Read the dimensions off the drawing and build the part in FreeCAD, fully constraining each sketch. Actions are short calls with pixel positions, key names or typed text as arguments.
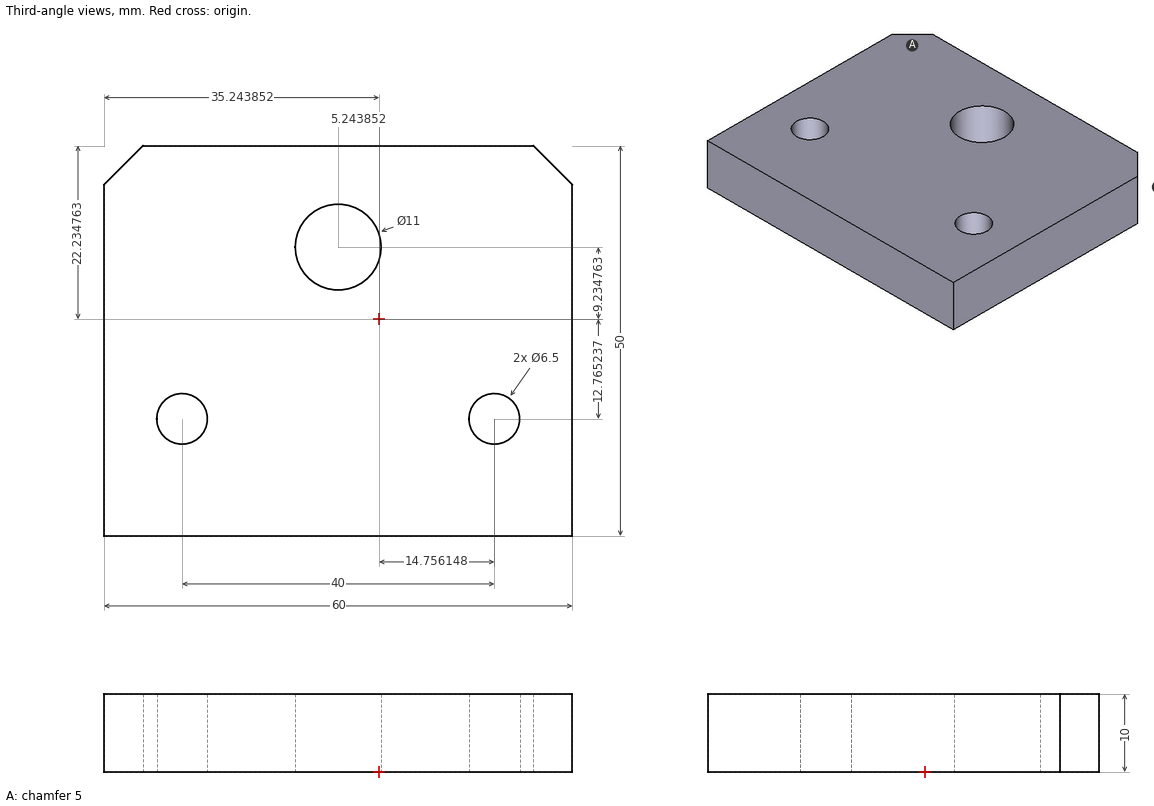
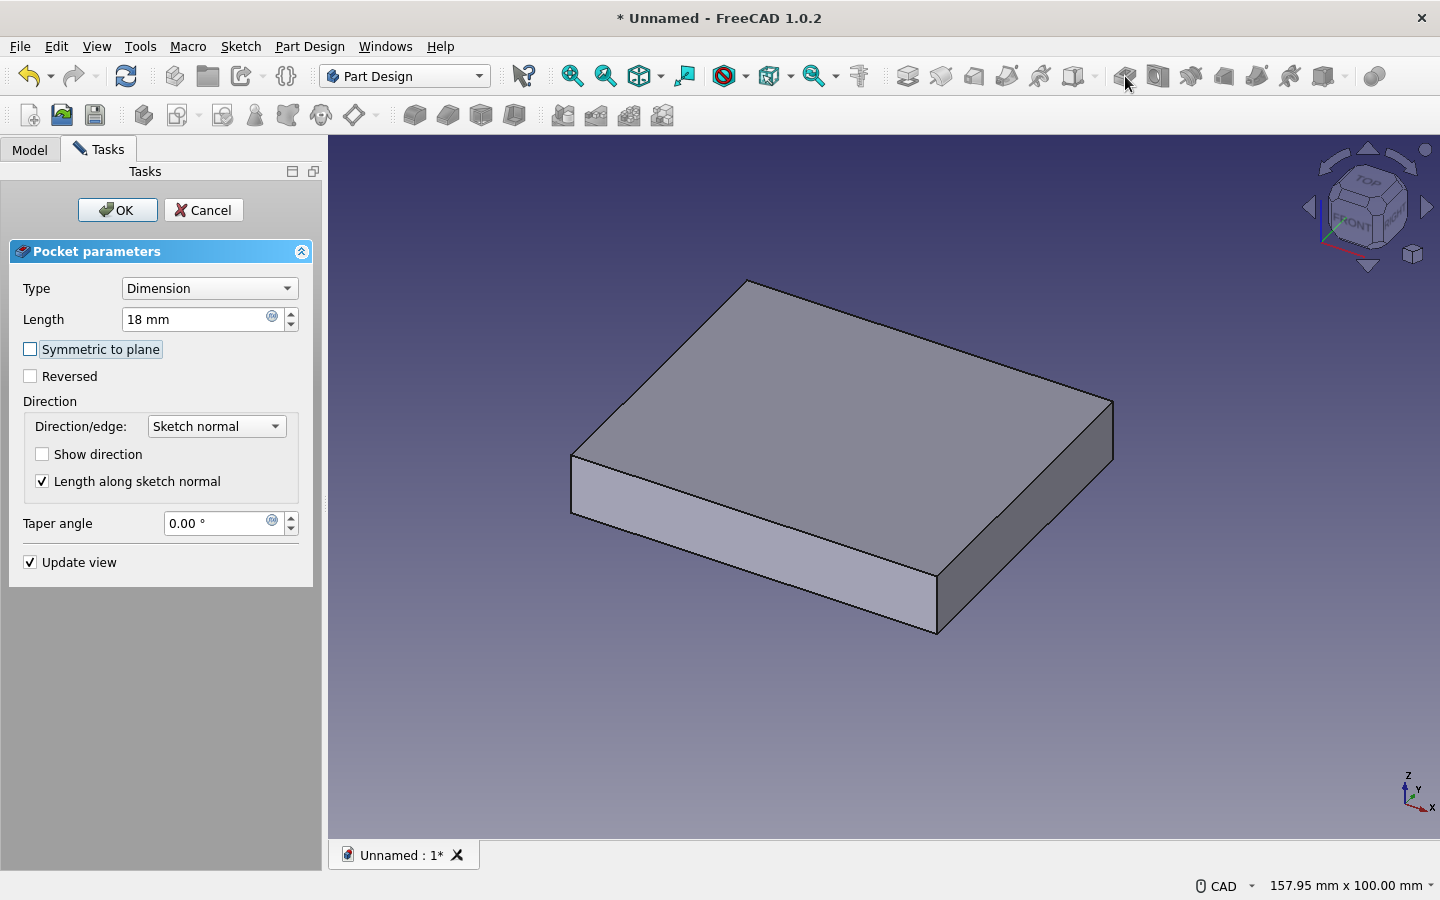
click(31, 376)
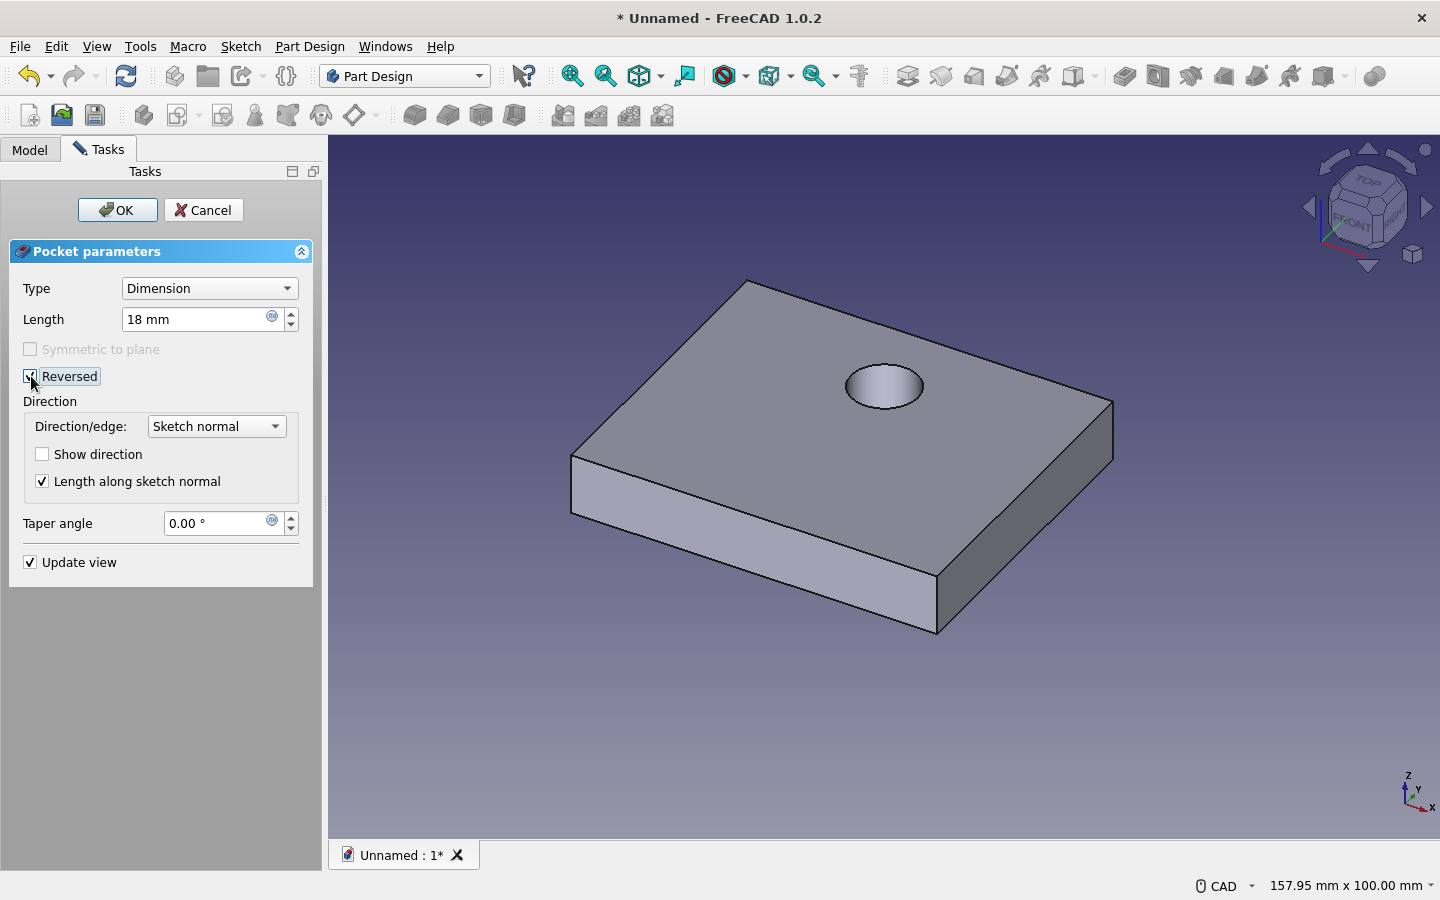
click(118, 210)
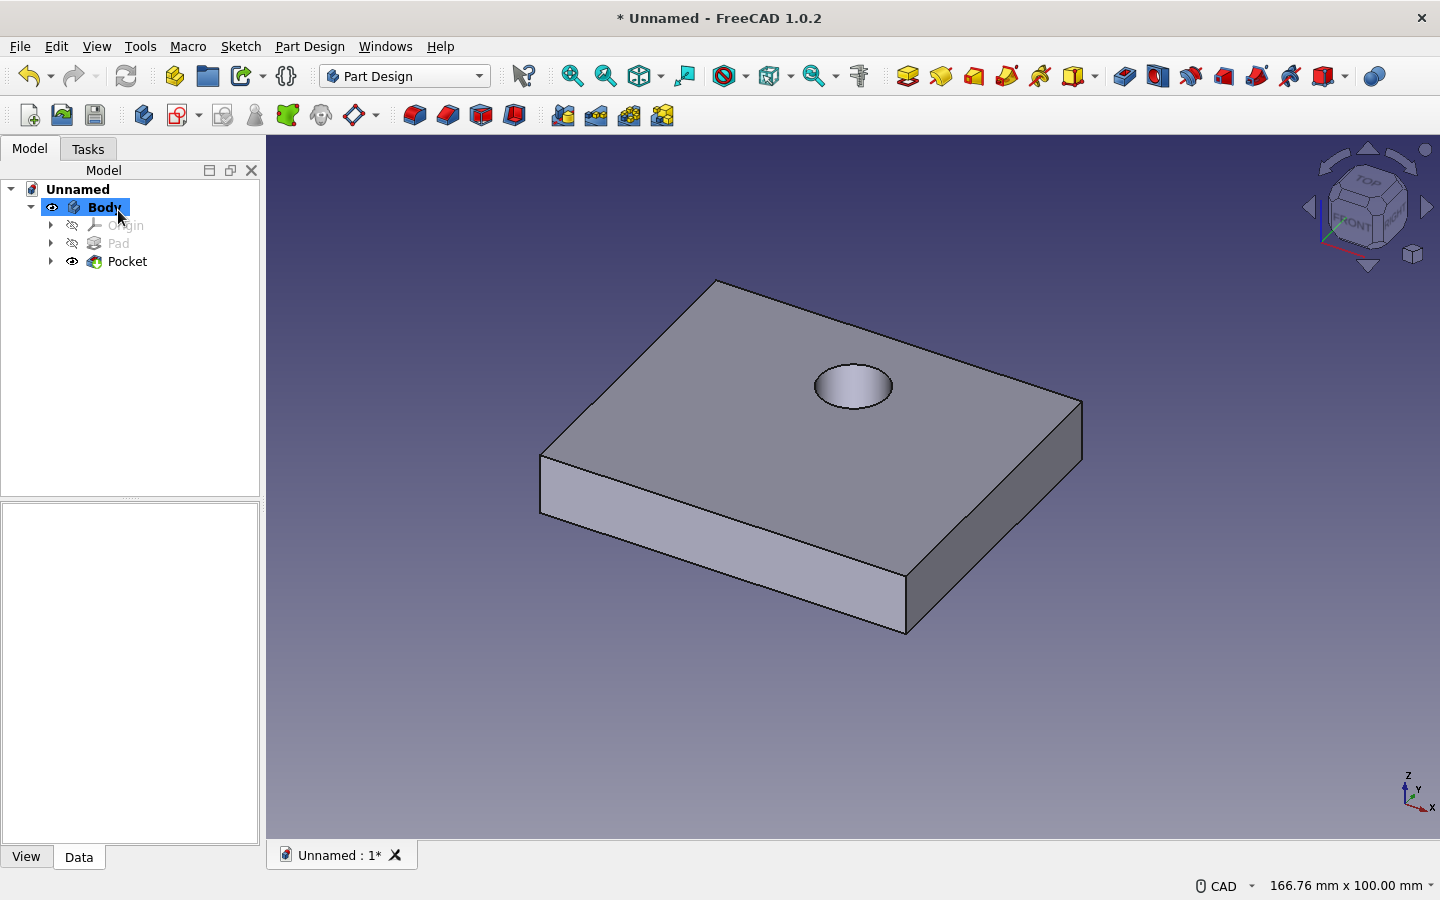
key(0)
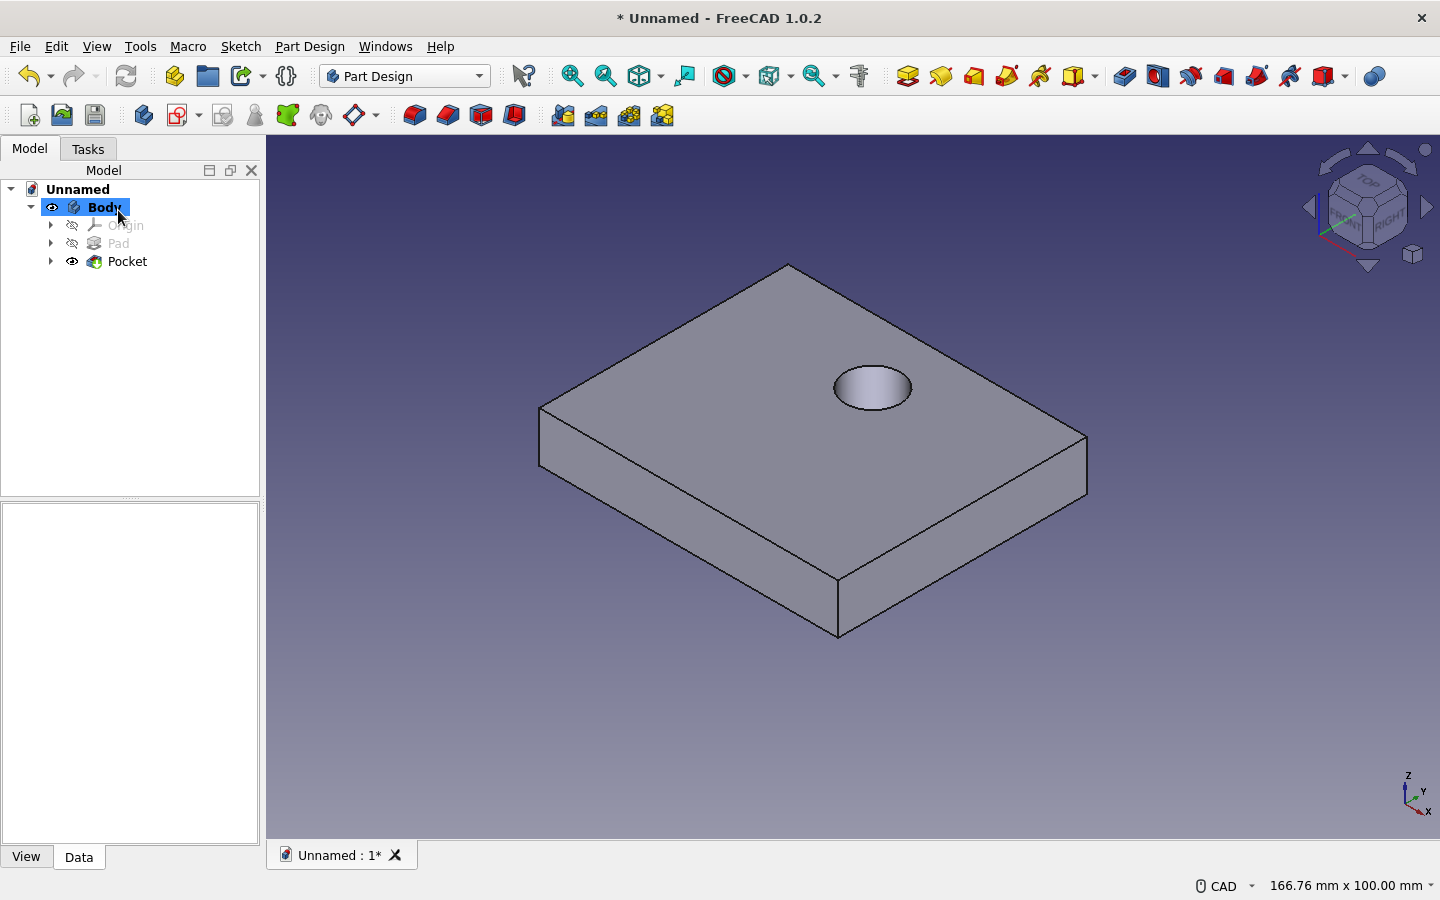
key(2)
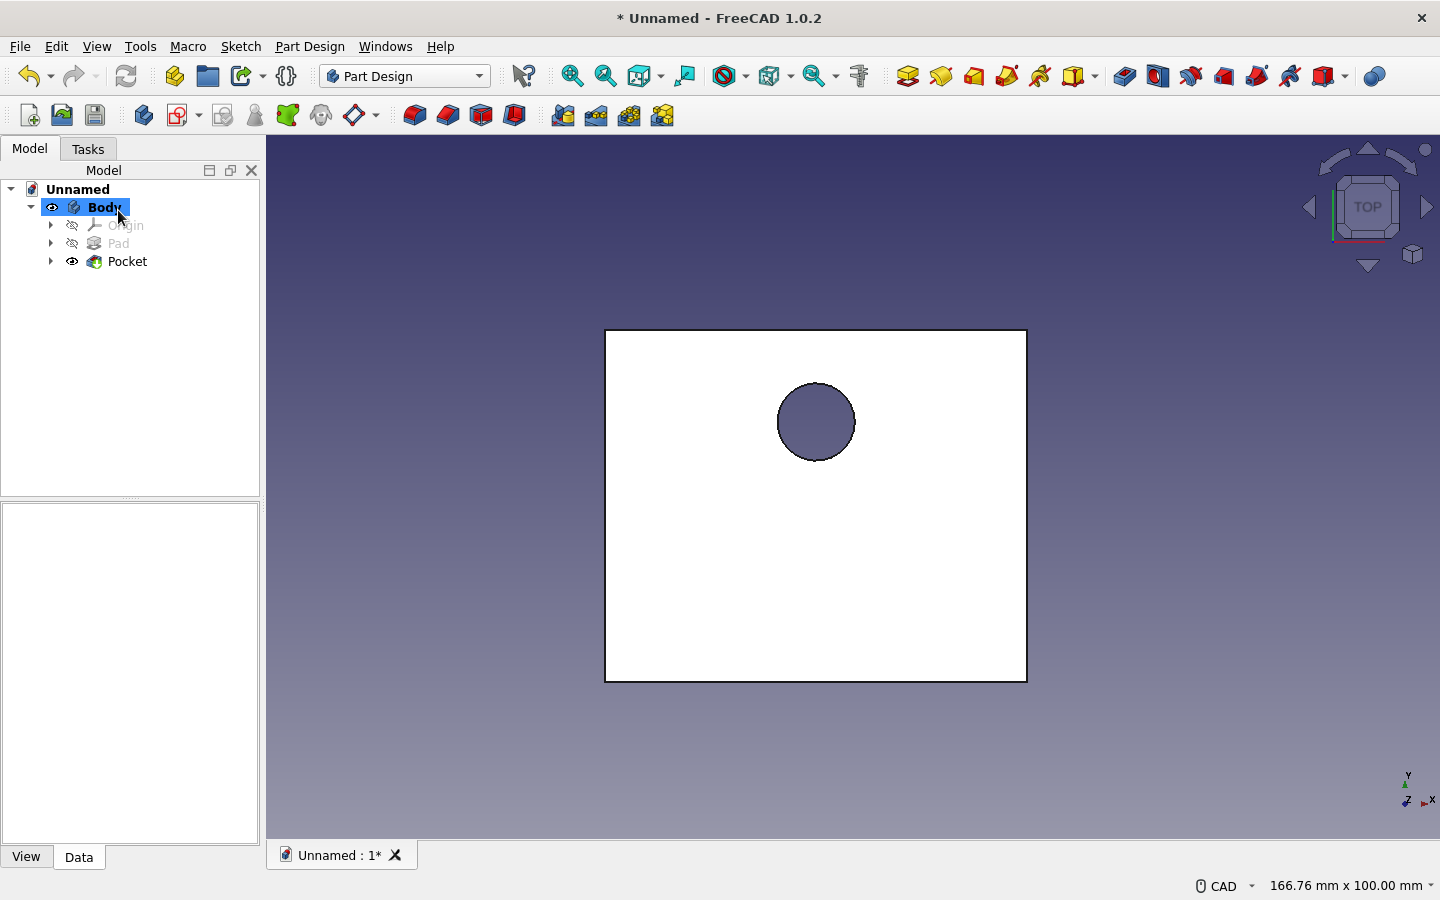
key(1)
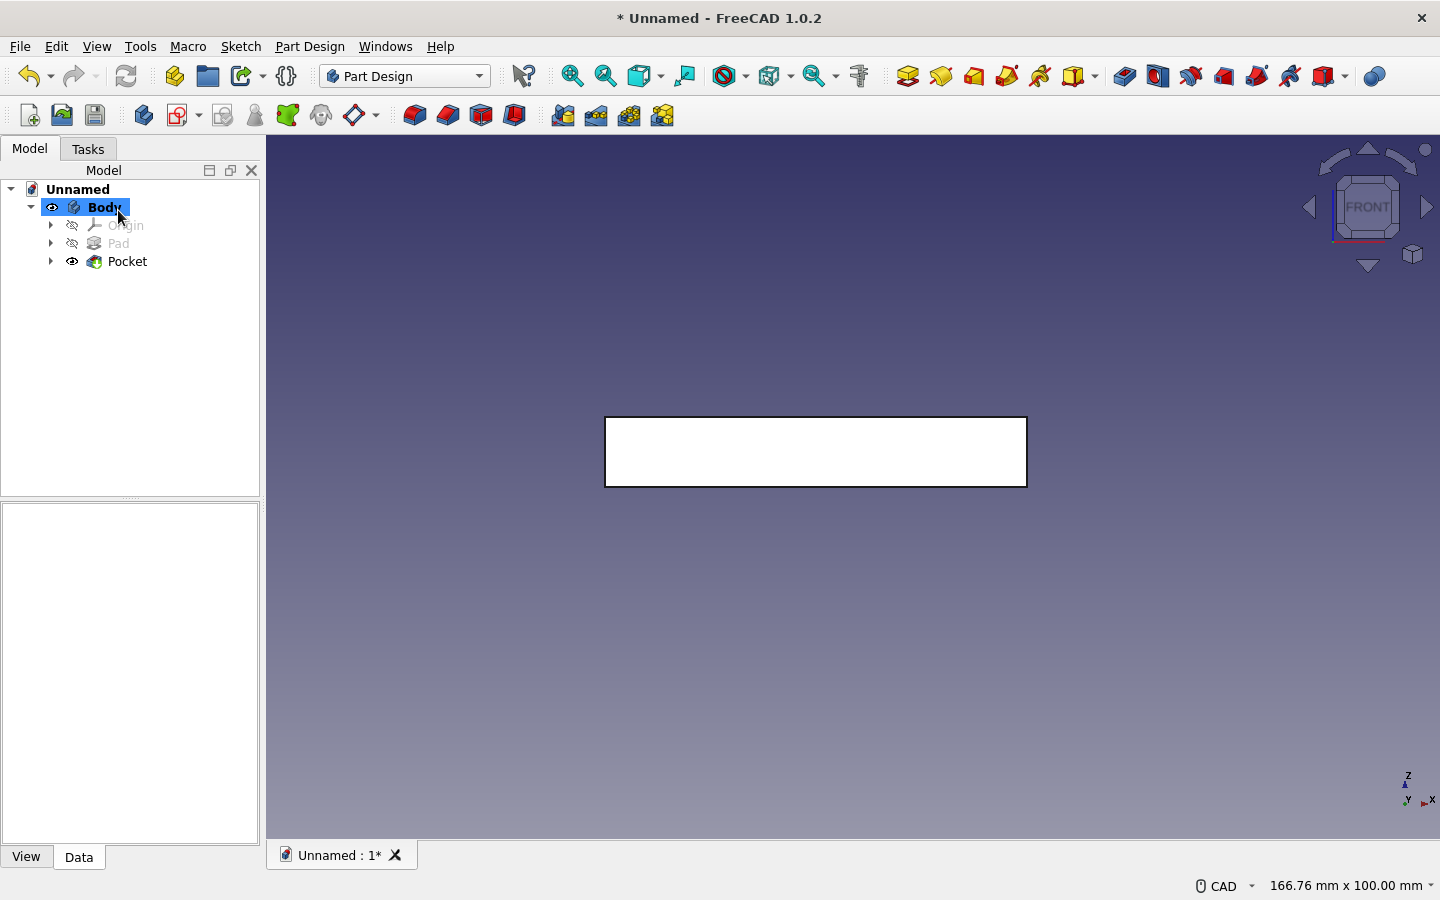
click(573, 76)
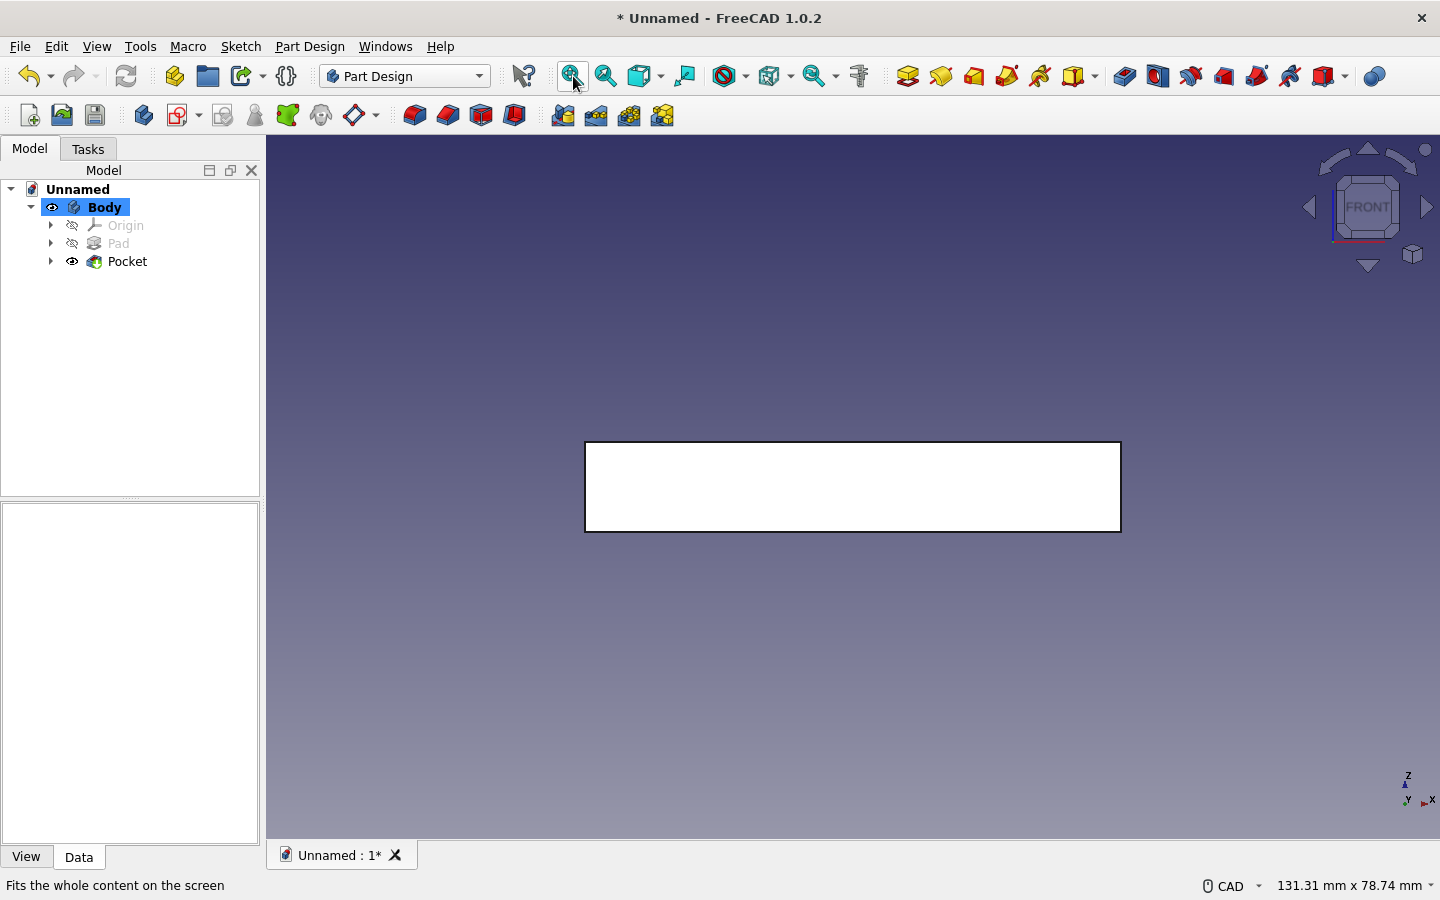
key(3)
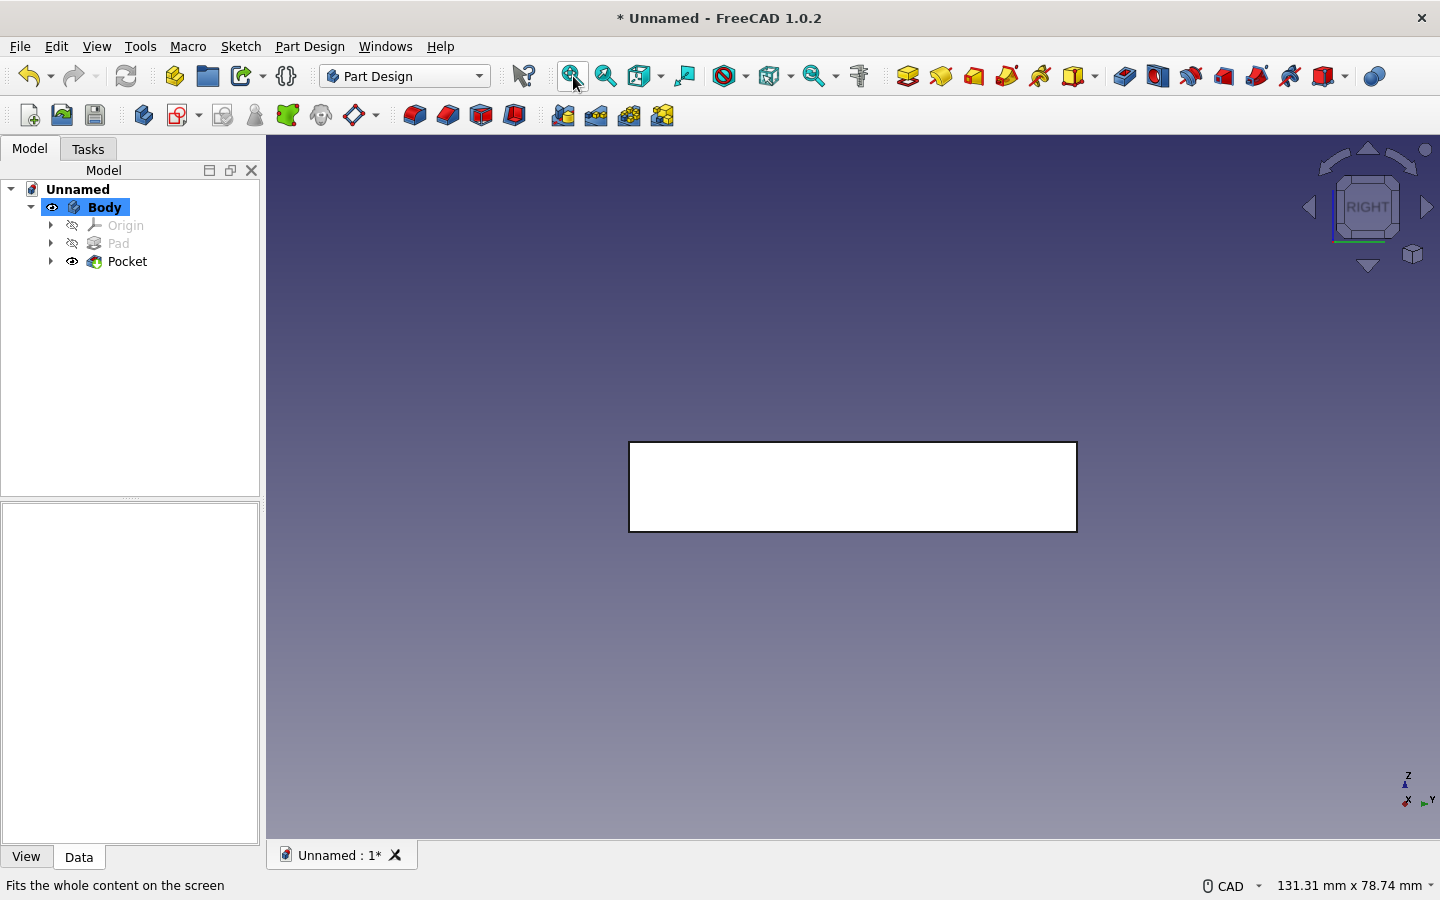
click(573, 76)